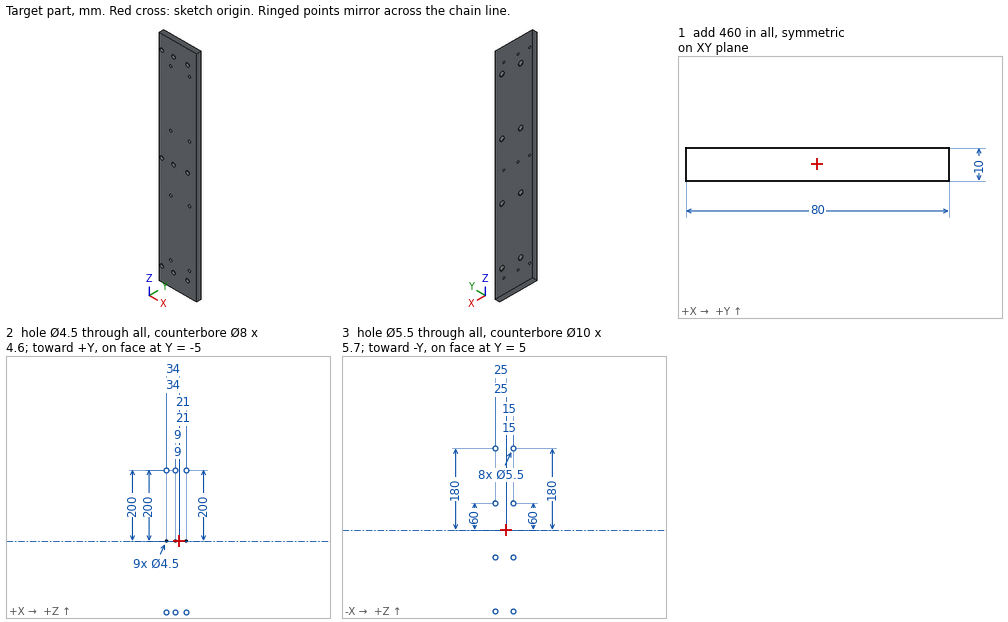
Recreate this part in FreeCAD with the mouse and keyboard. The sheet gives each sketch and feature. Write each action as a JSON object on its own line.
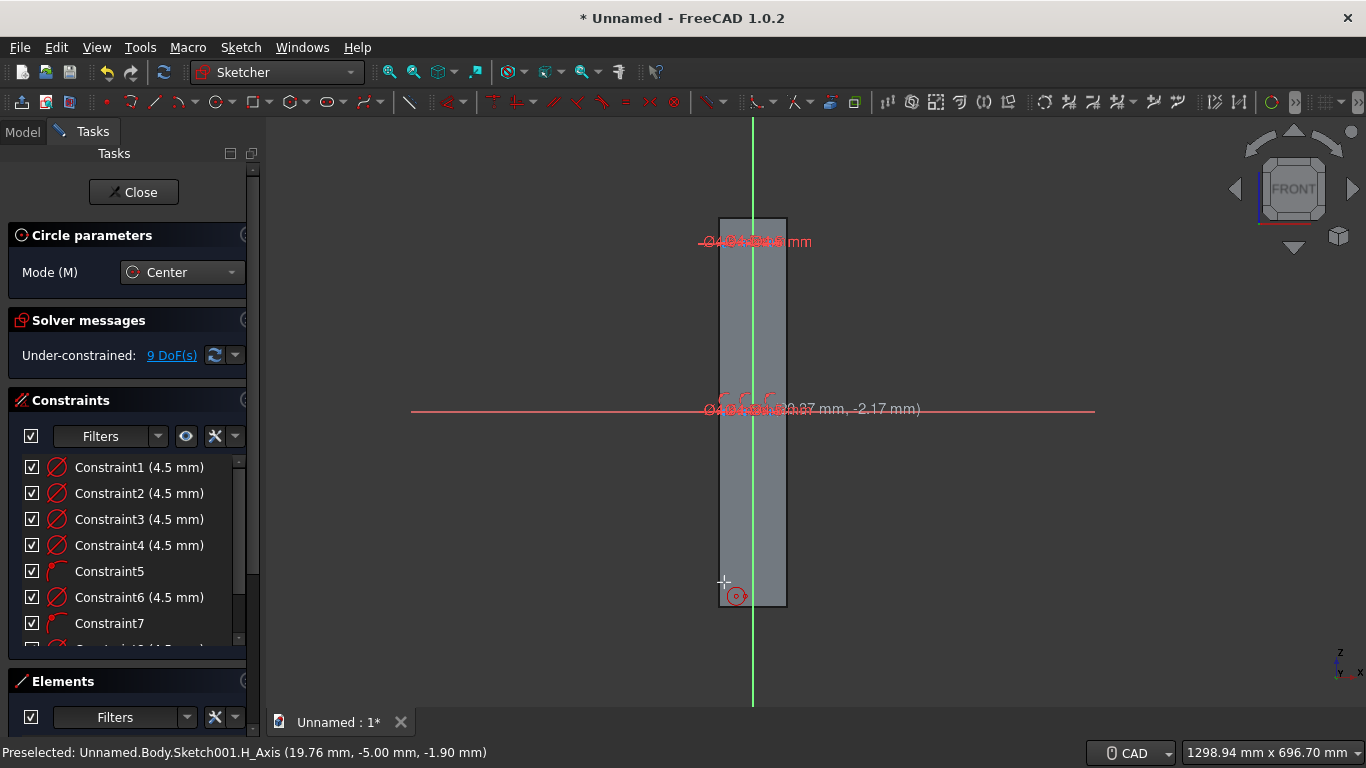
{"action": "left_click", "coordinate": [724, 582]}
{"action": "mouse_move", "coordinate": [726, 580]}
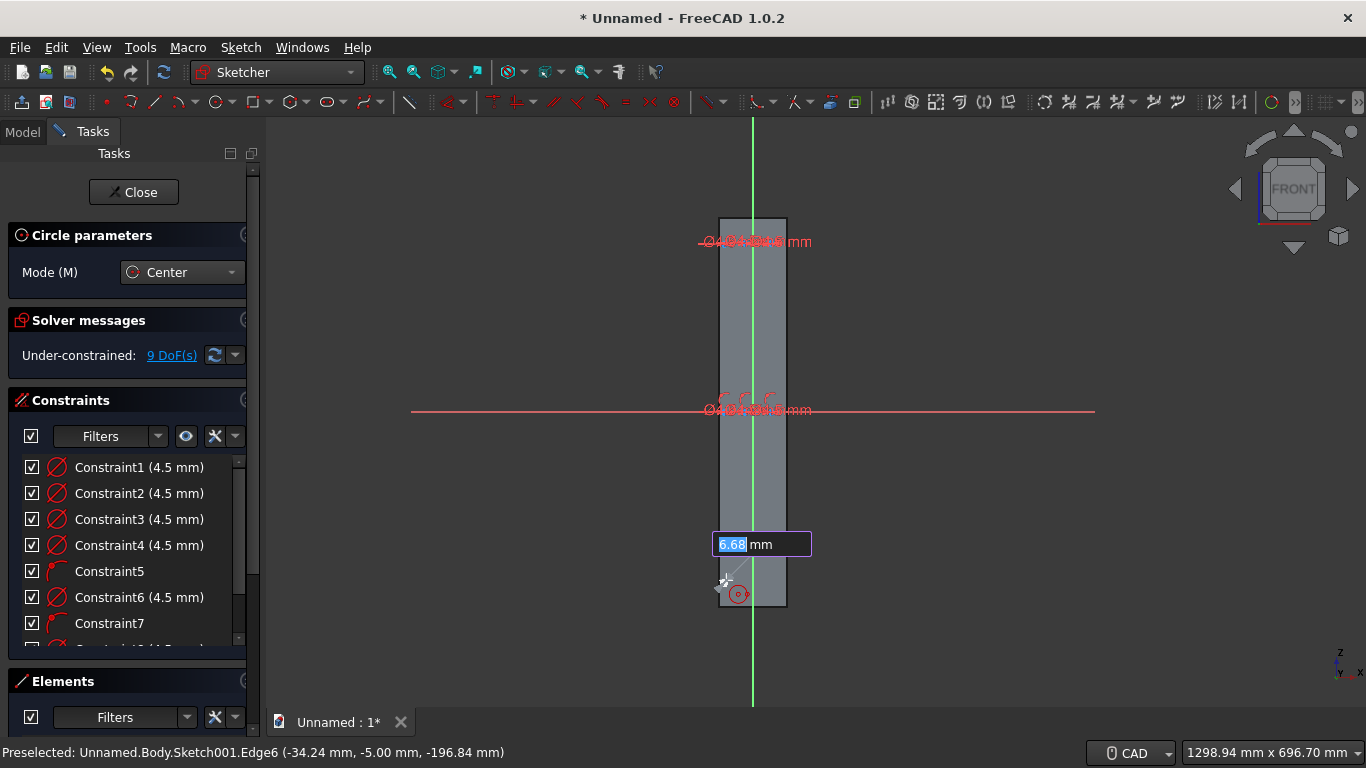
{"action": "type", "text": "4.5"}
{"action": "key", "text": "Return"}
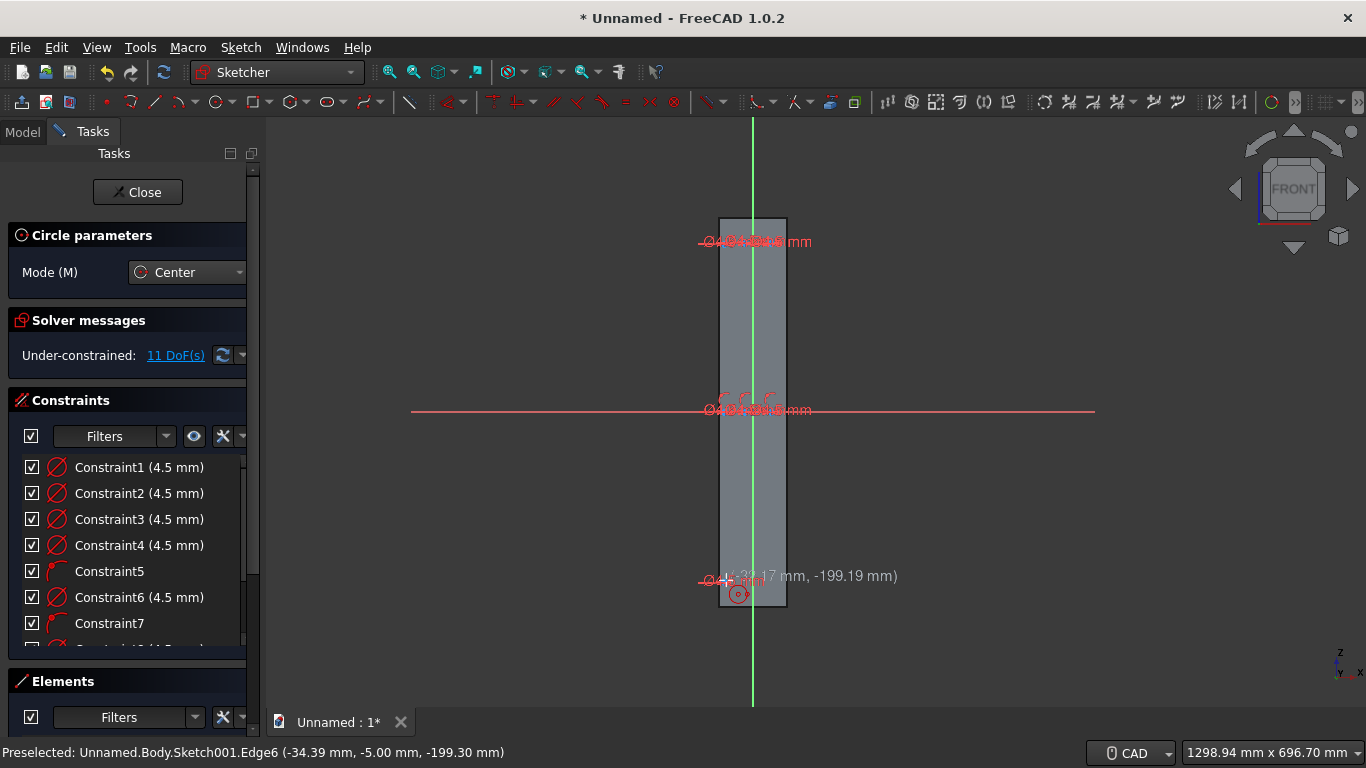
{"action": "scroll", "coordinate": [746, 582], "scroll_direction": "up", "scroll_amount": 13}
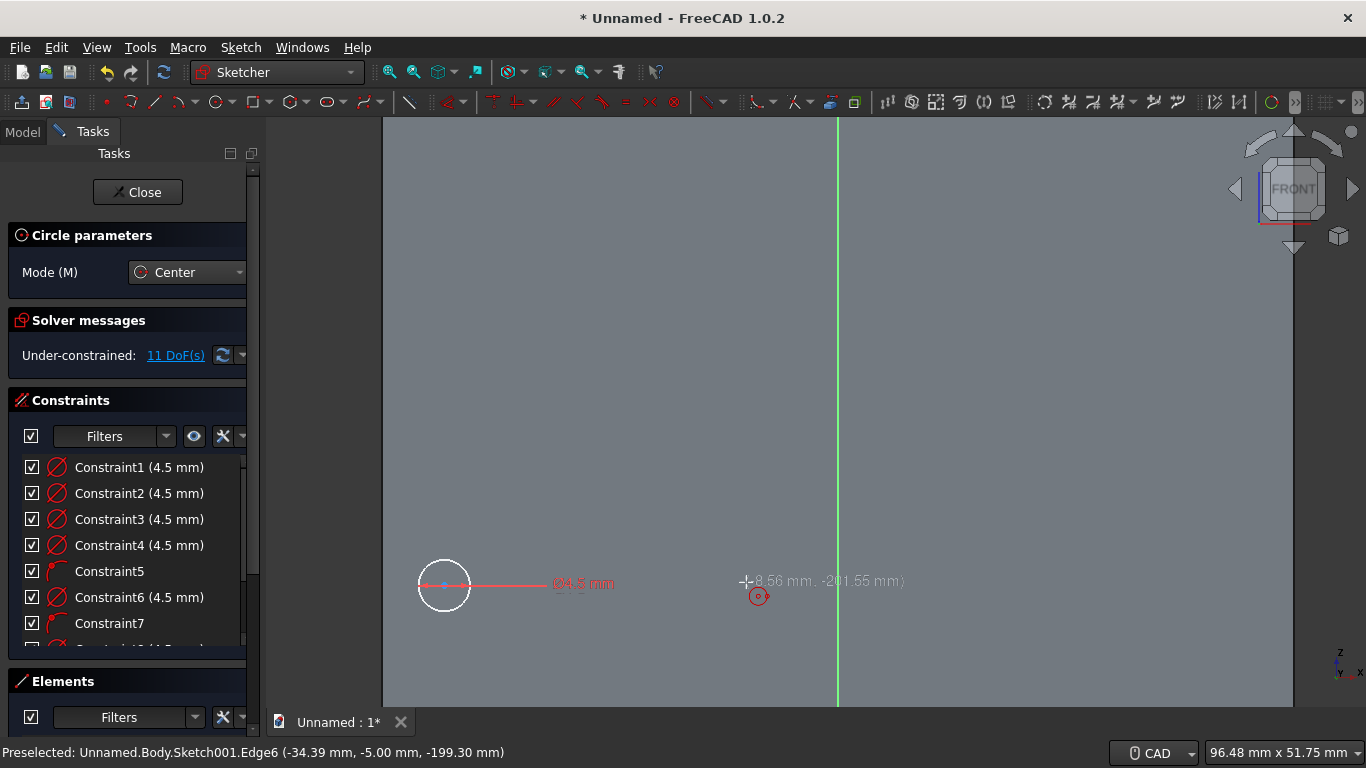
{"action": "scroll", "coordinate": [746, 582], "scroll_direction": "down", "scroll_amount": 13}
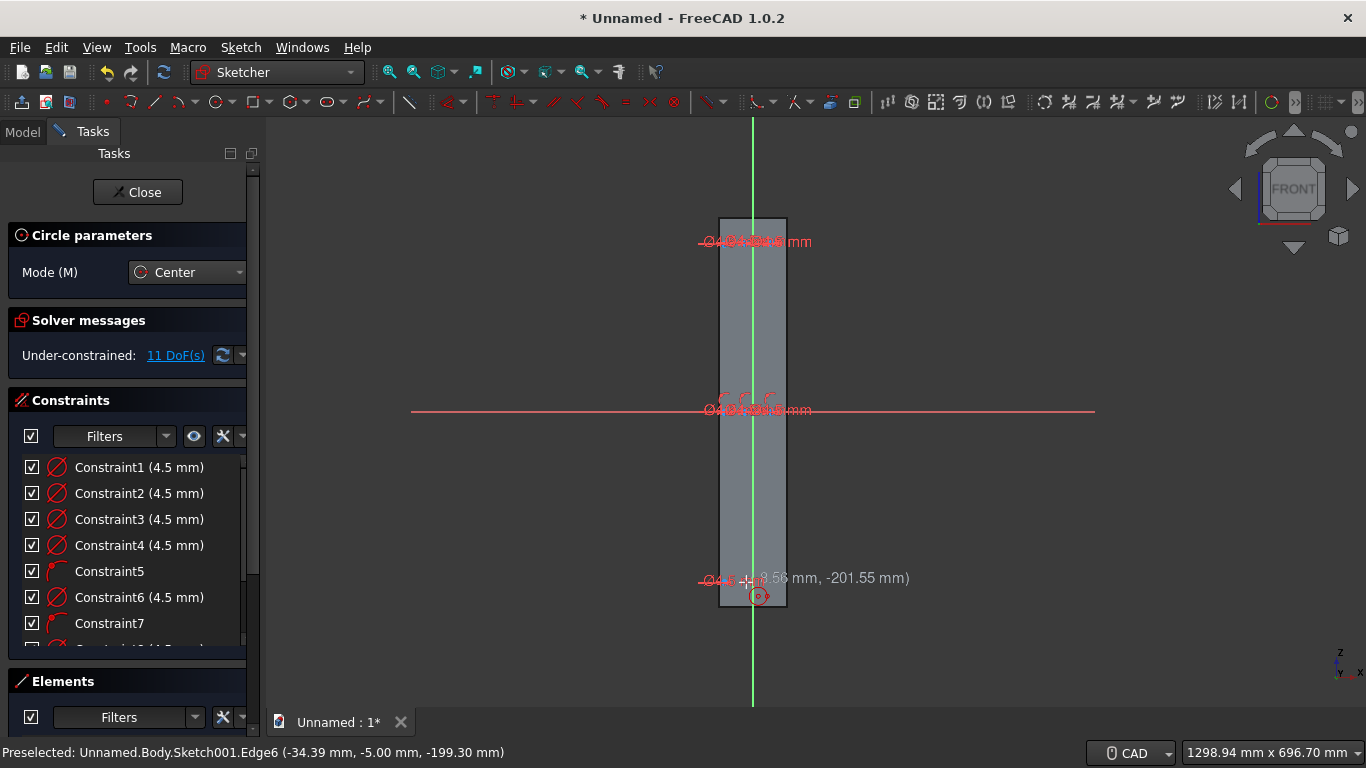
{"action": "scroll", "coordinate": [746, 582], "scroll_direction": "up", "scroll_amount": 4}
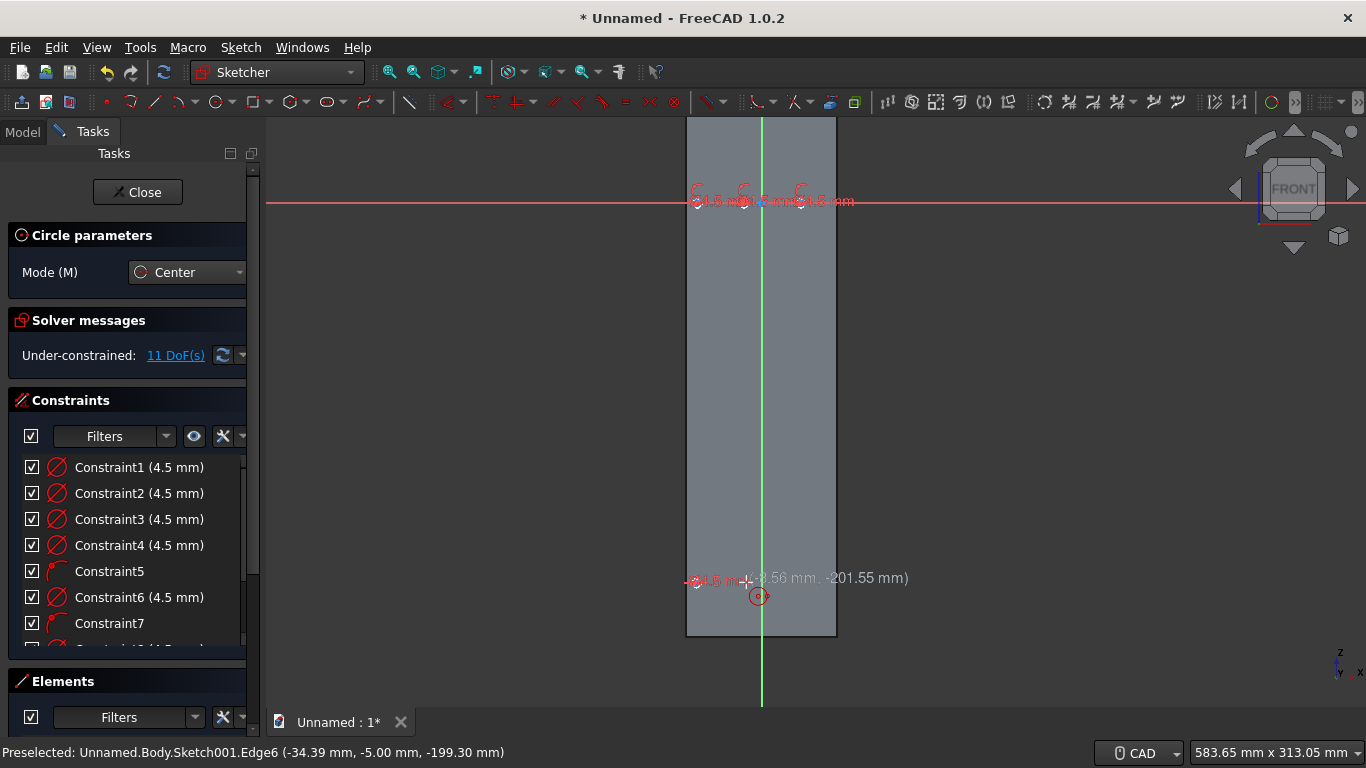
{"action": "left_click", "coordinate": [745, 580]}
{"action": "mouse_move", "coordinate": [742, 577]}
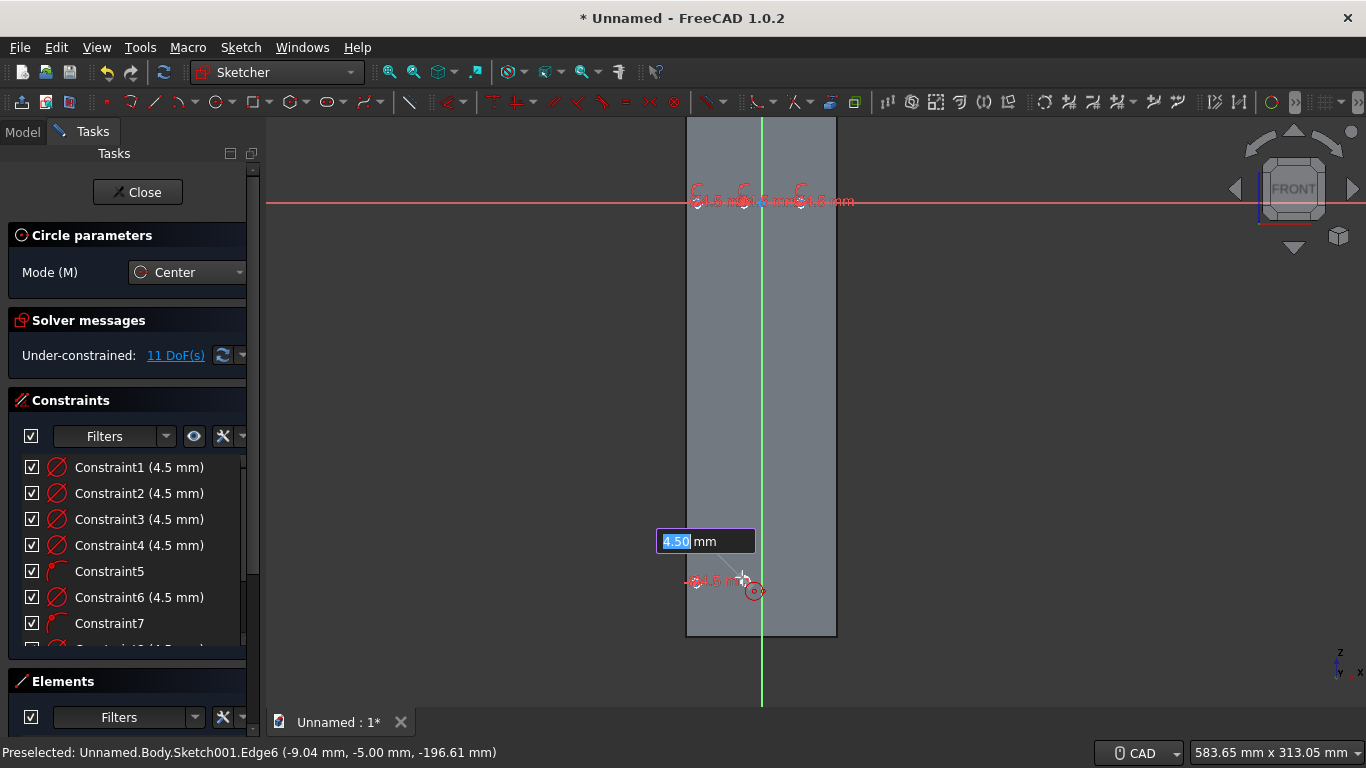
{"action": "type", "text": "4.5"}
{"action": "key", "text": "Return"}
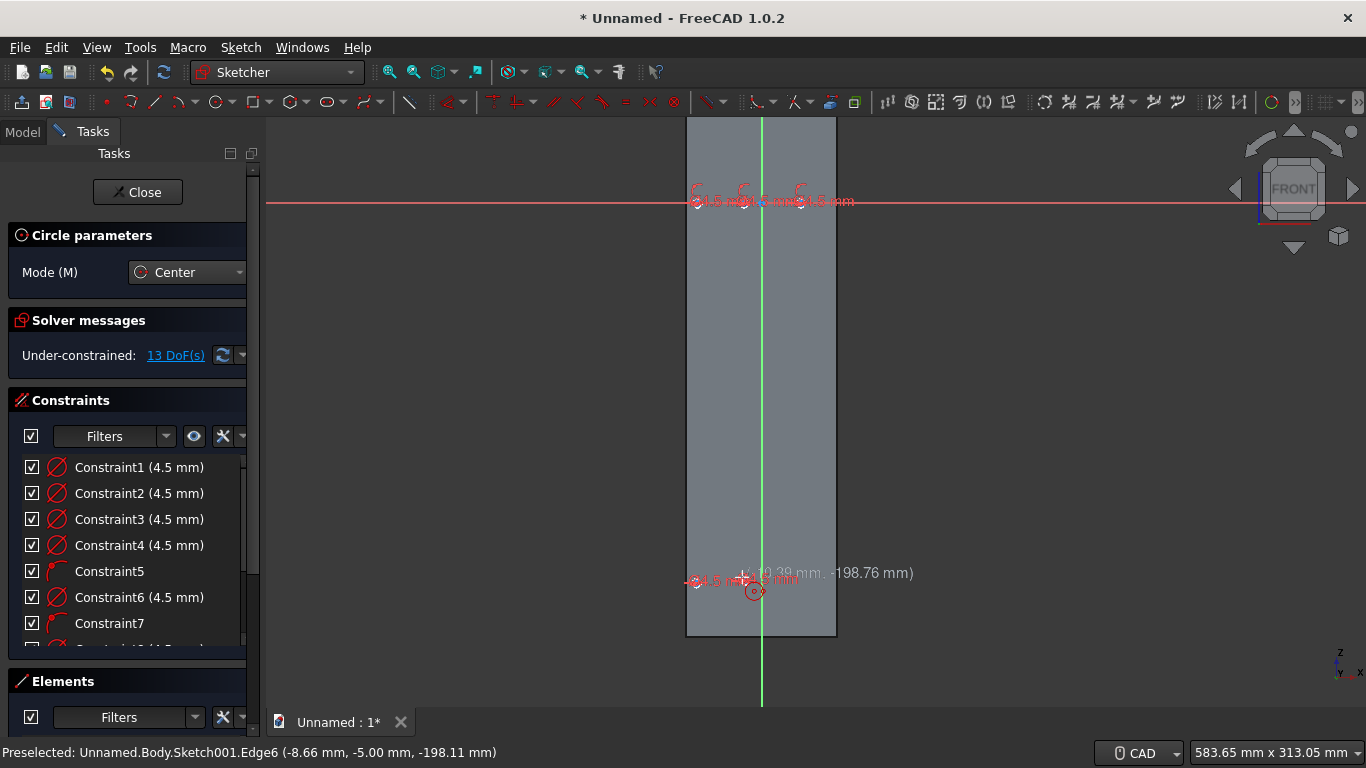
{"action": "scroll", "coordinate": [801, 580], "scroll_direction": "up", "scroll_amount": 9}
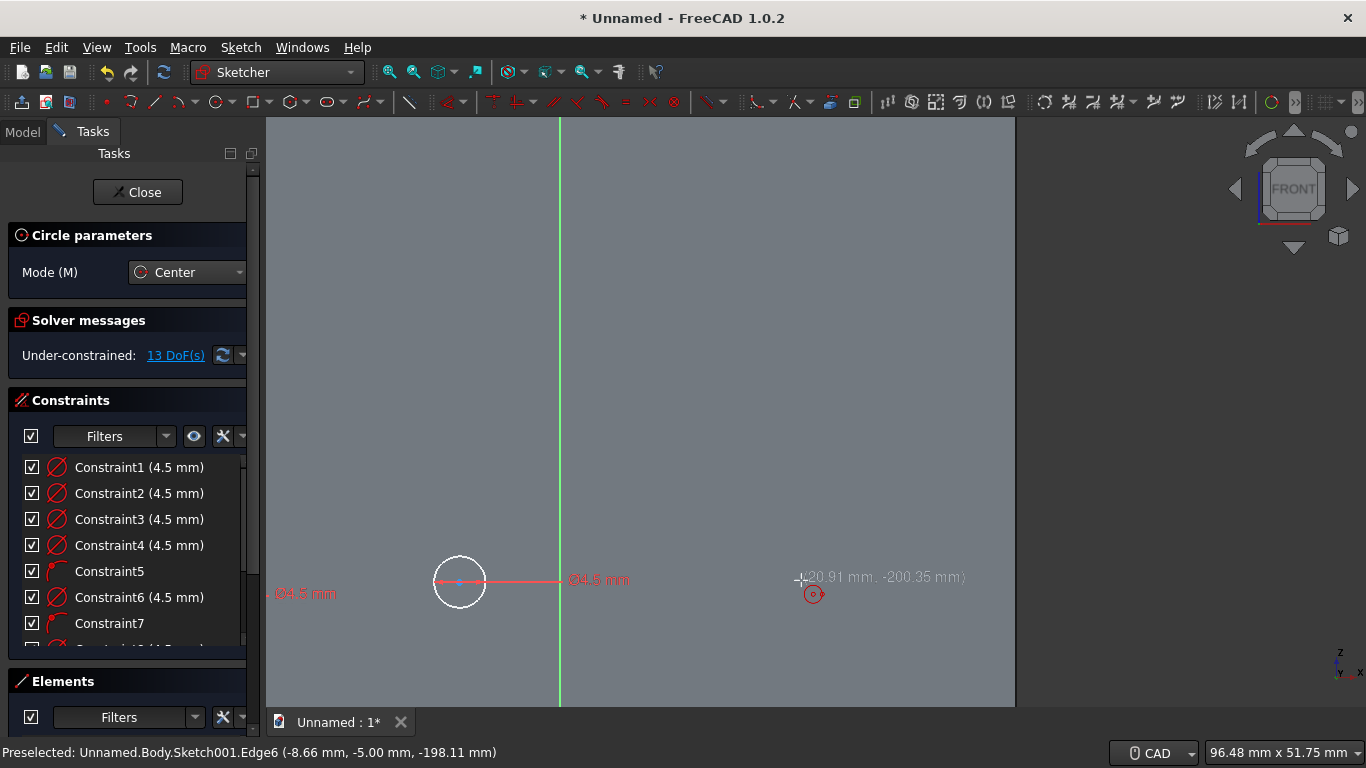
{"action": "scroll", "coordinate": [768, 582], "scroll_direction": "down", "scroll_amount": 13}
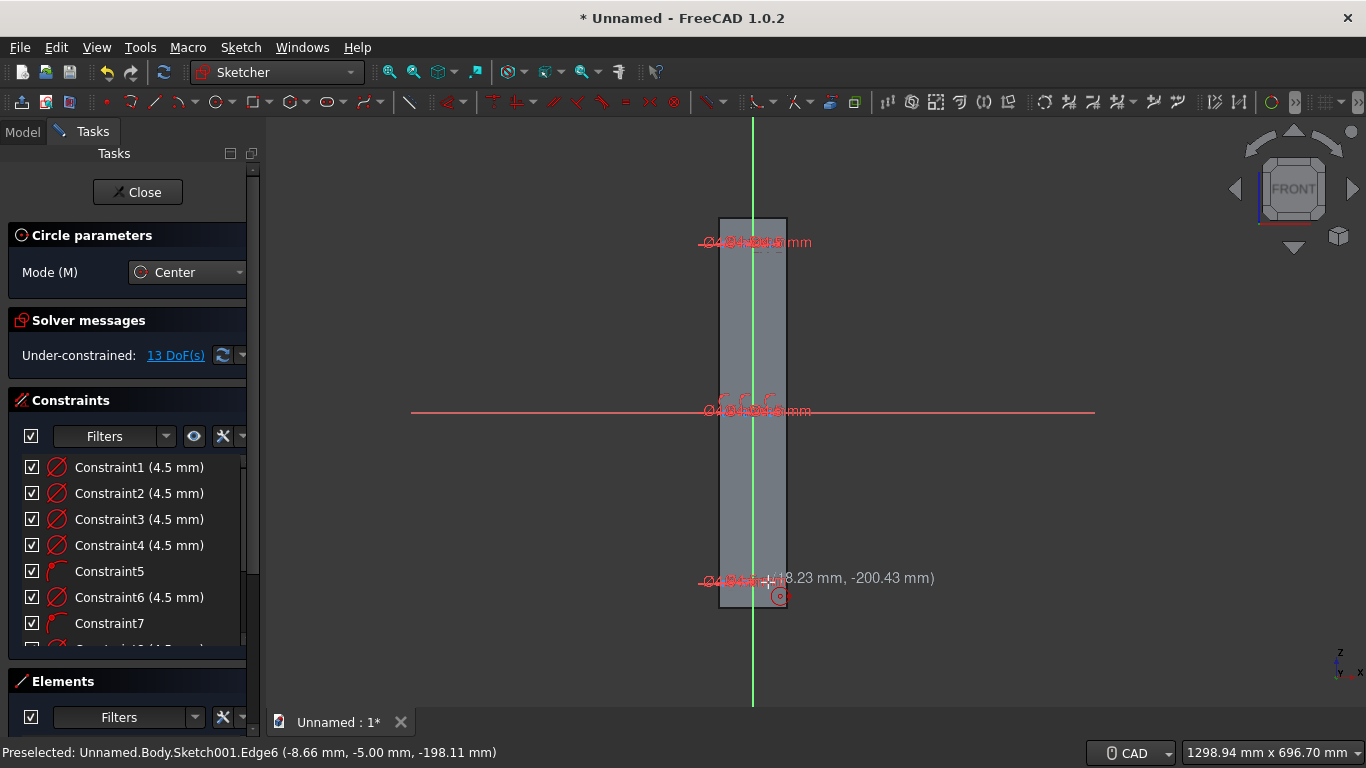
{"action": "left_click", "coordinate": [771, 582]}
{"action": "mouse_move", "coordinate": [772, 581]}